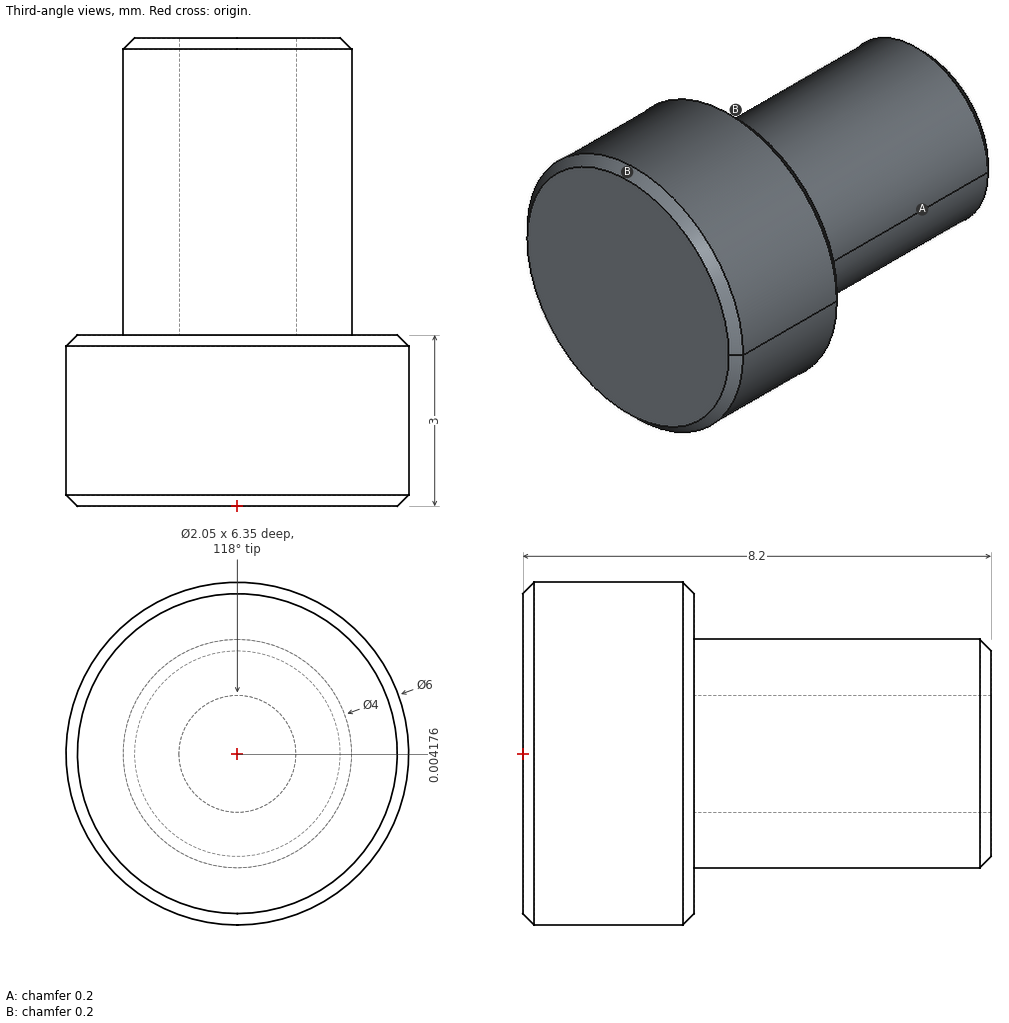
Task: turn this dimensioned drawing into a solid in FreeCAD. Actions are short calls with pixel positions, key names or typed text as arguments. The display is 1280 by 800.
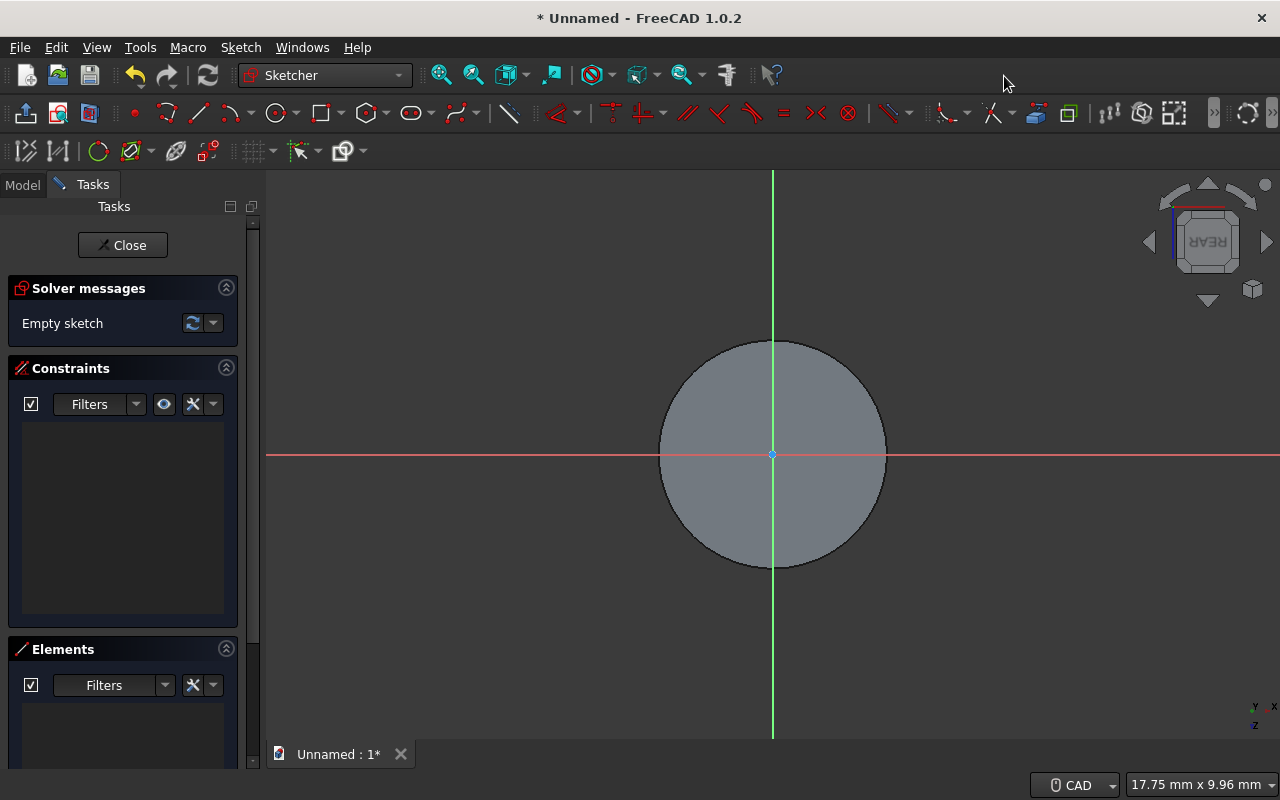
scroll(802, 454, up, 6)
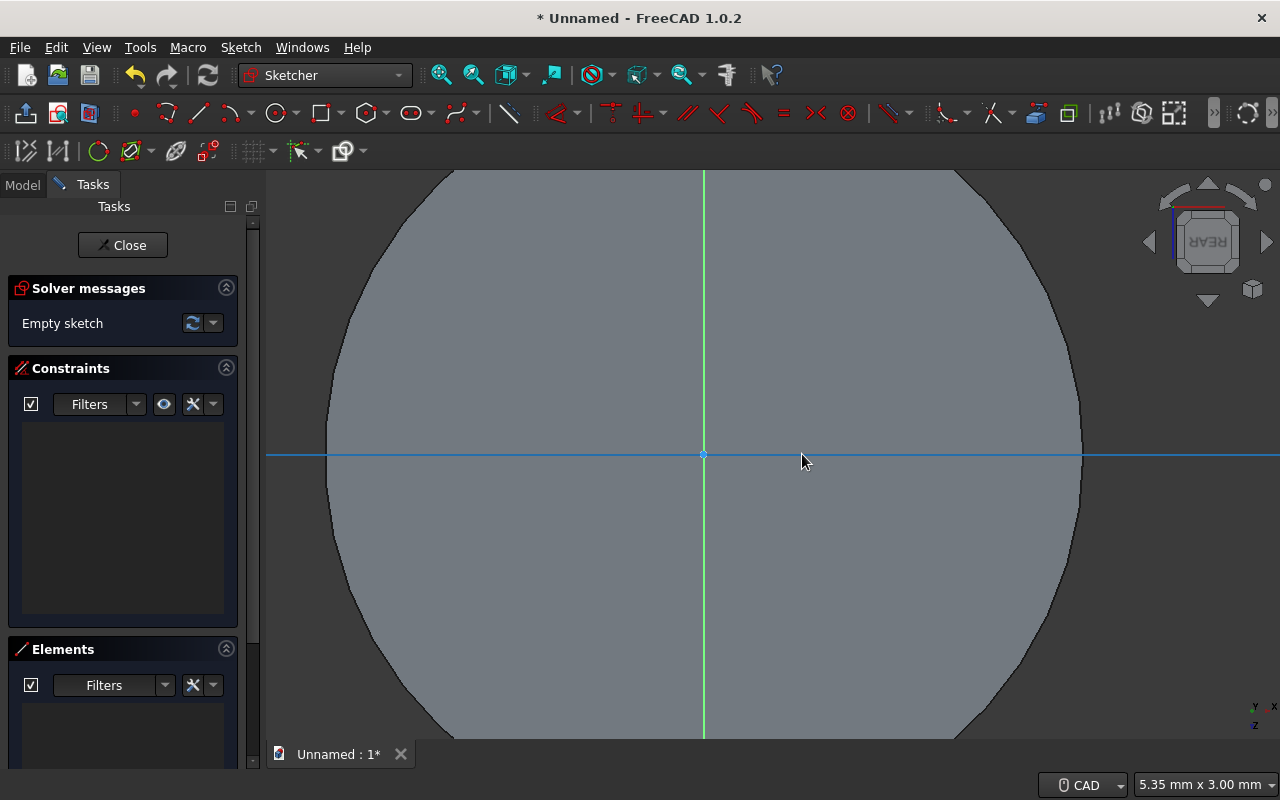
click(276, 114)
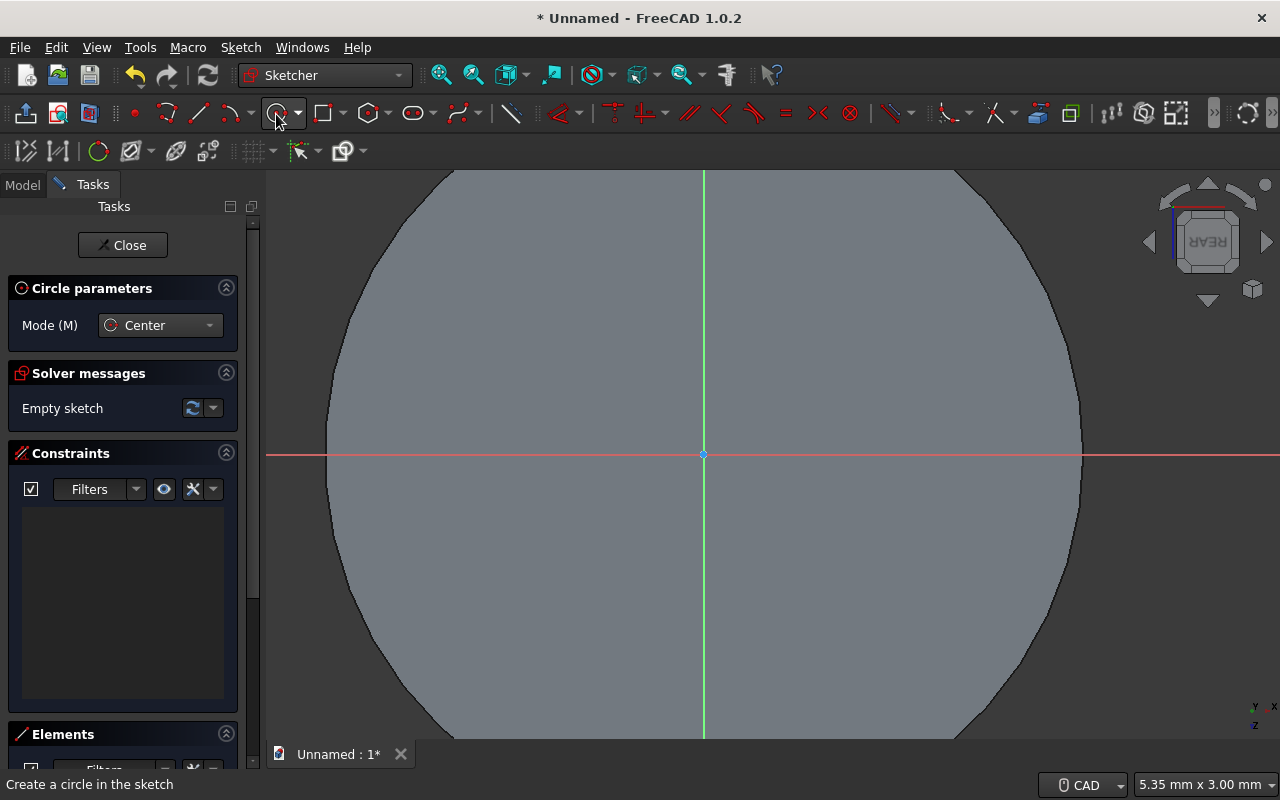
scroll(704, 454, up, 15)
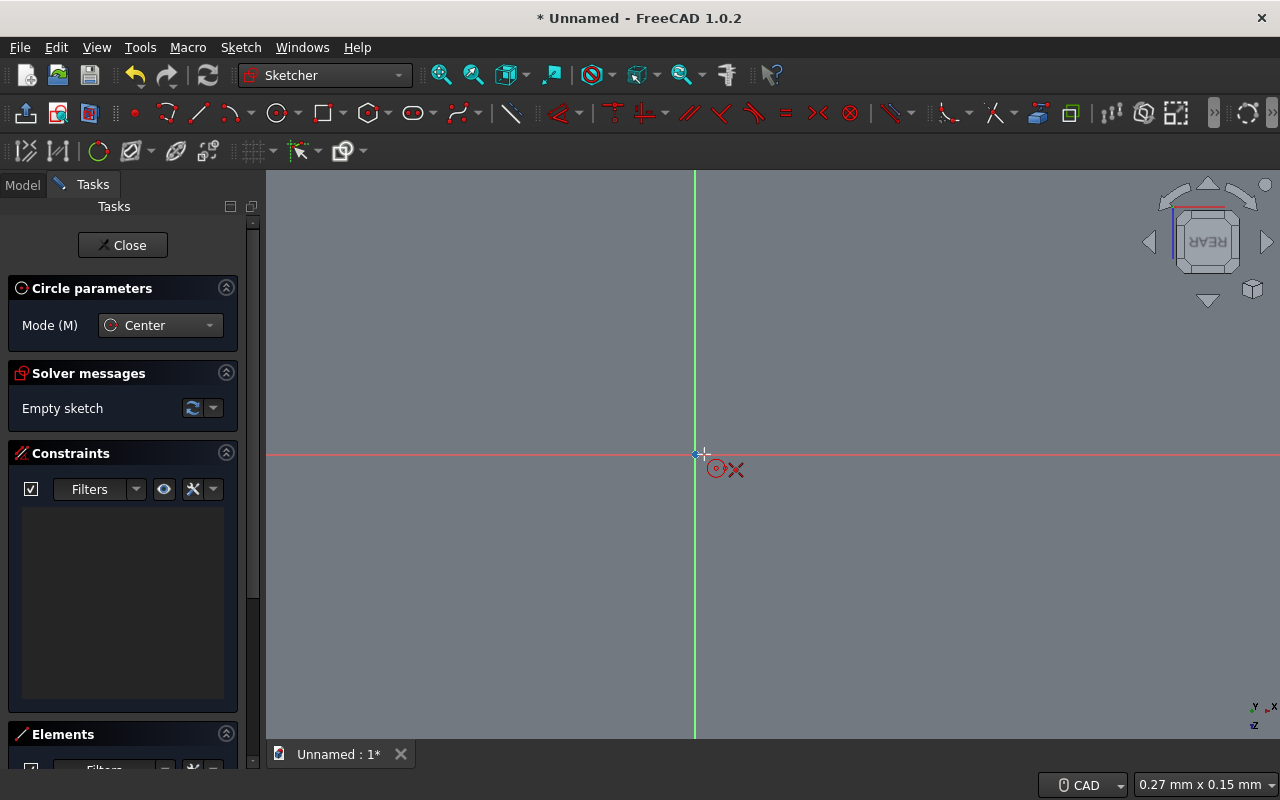
click(695, 439)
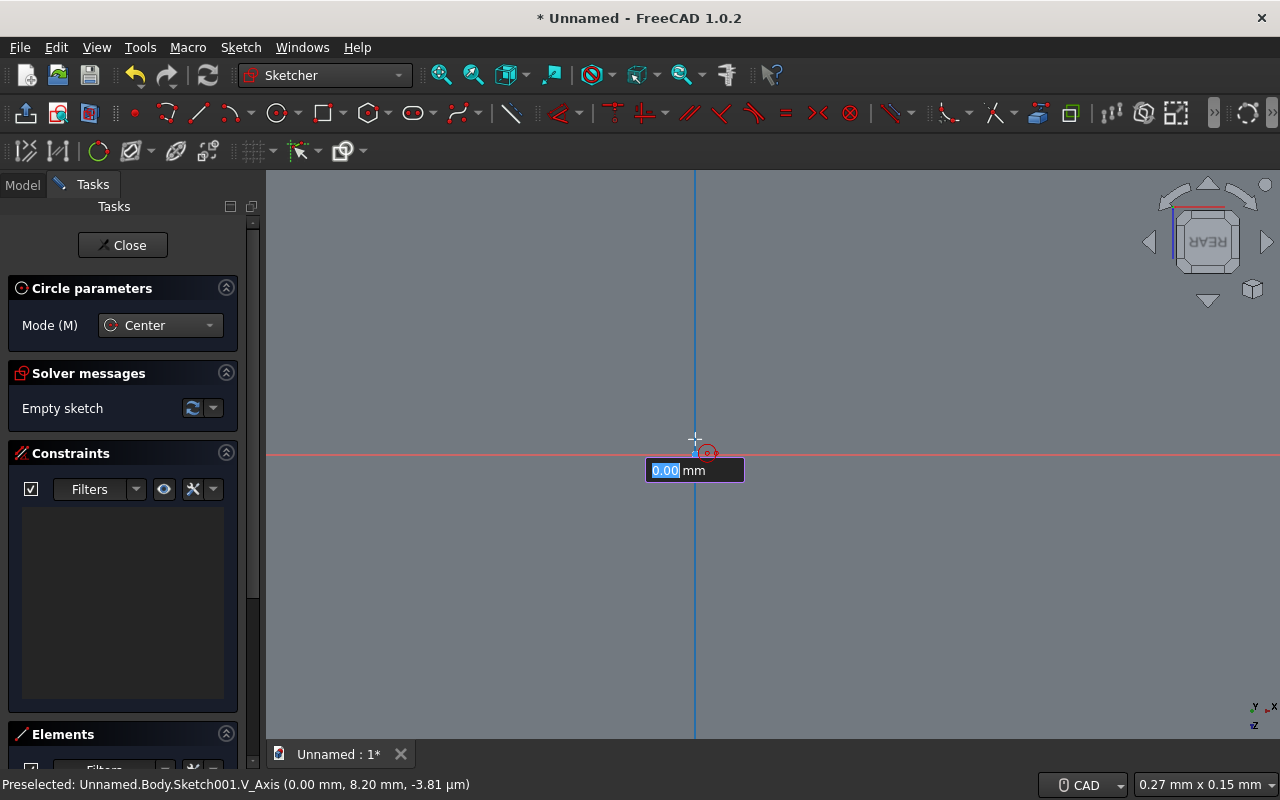
scroll(705, 455, down, 15)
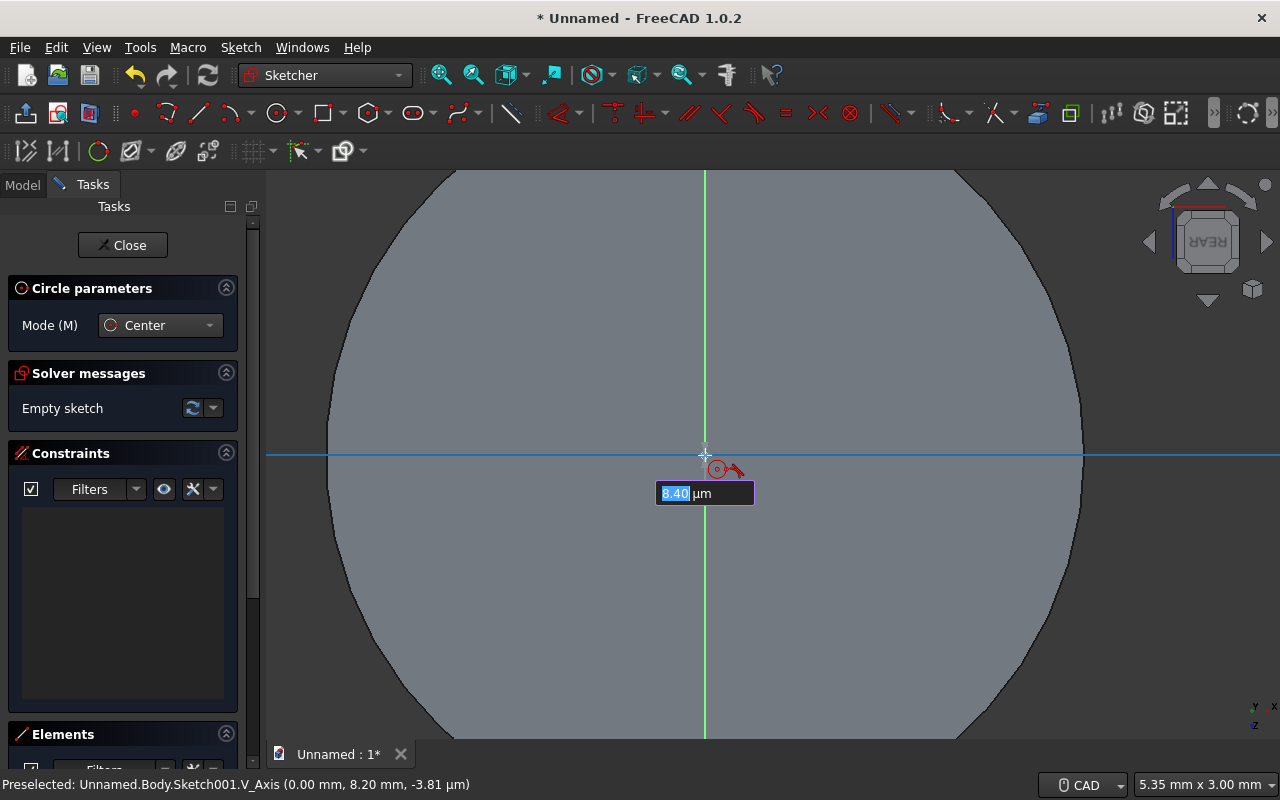
click(842, 317)
key(Escape)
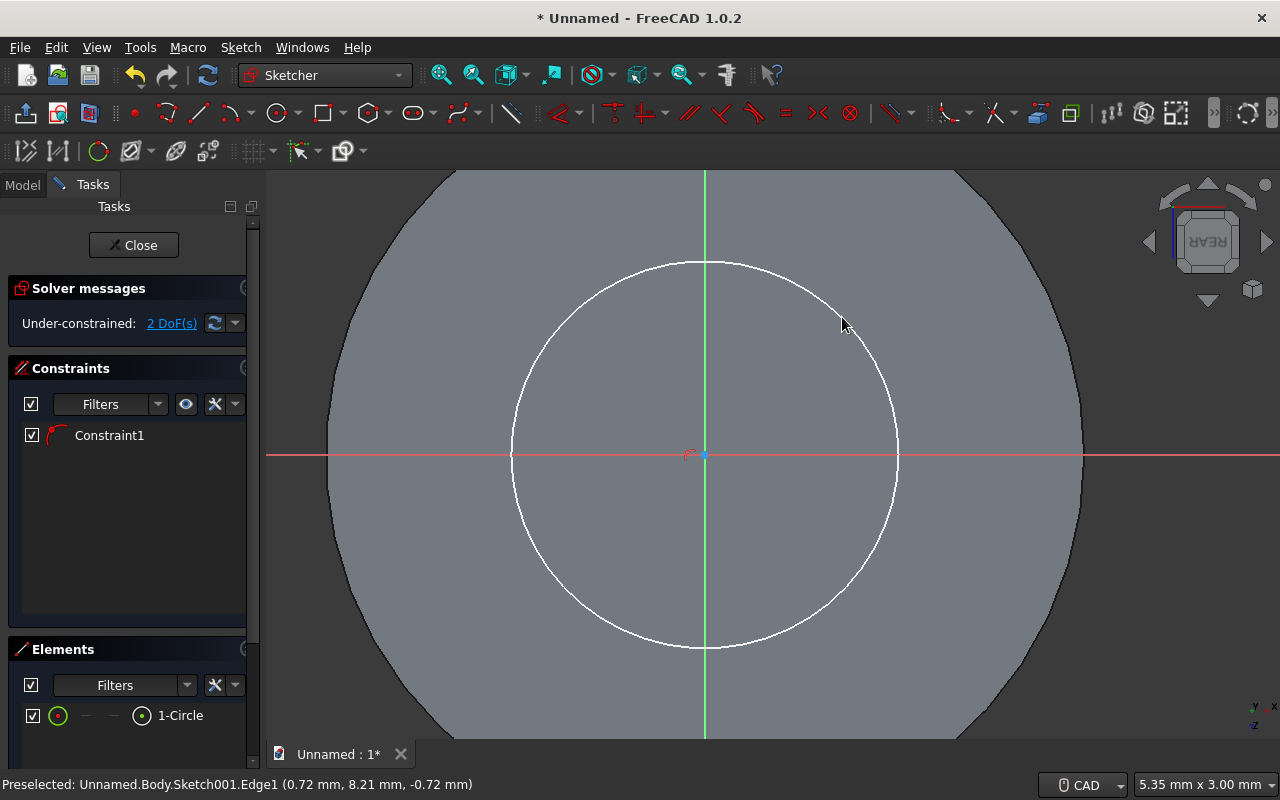
click(558, 114)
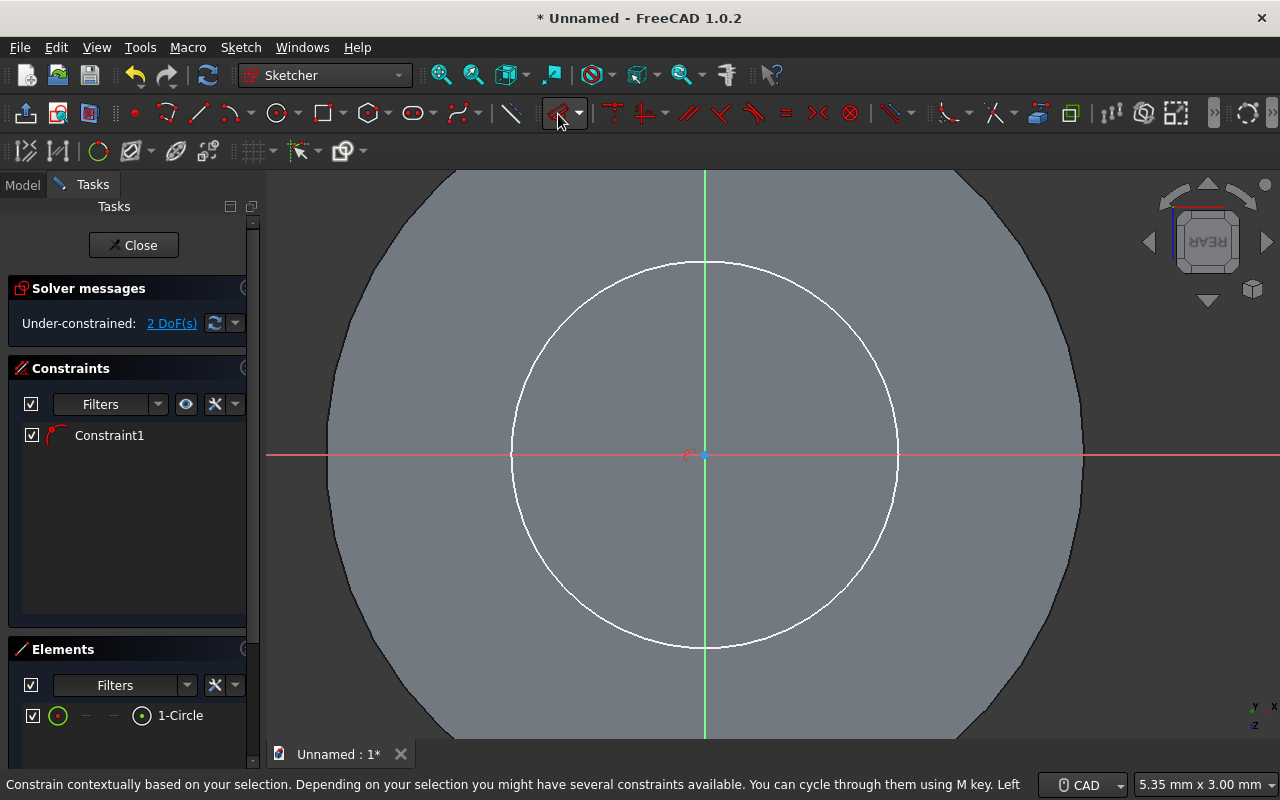
click(841, 317)
click(863, 294)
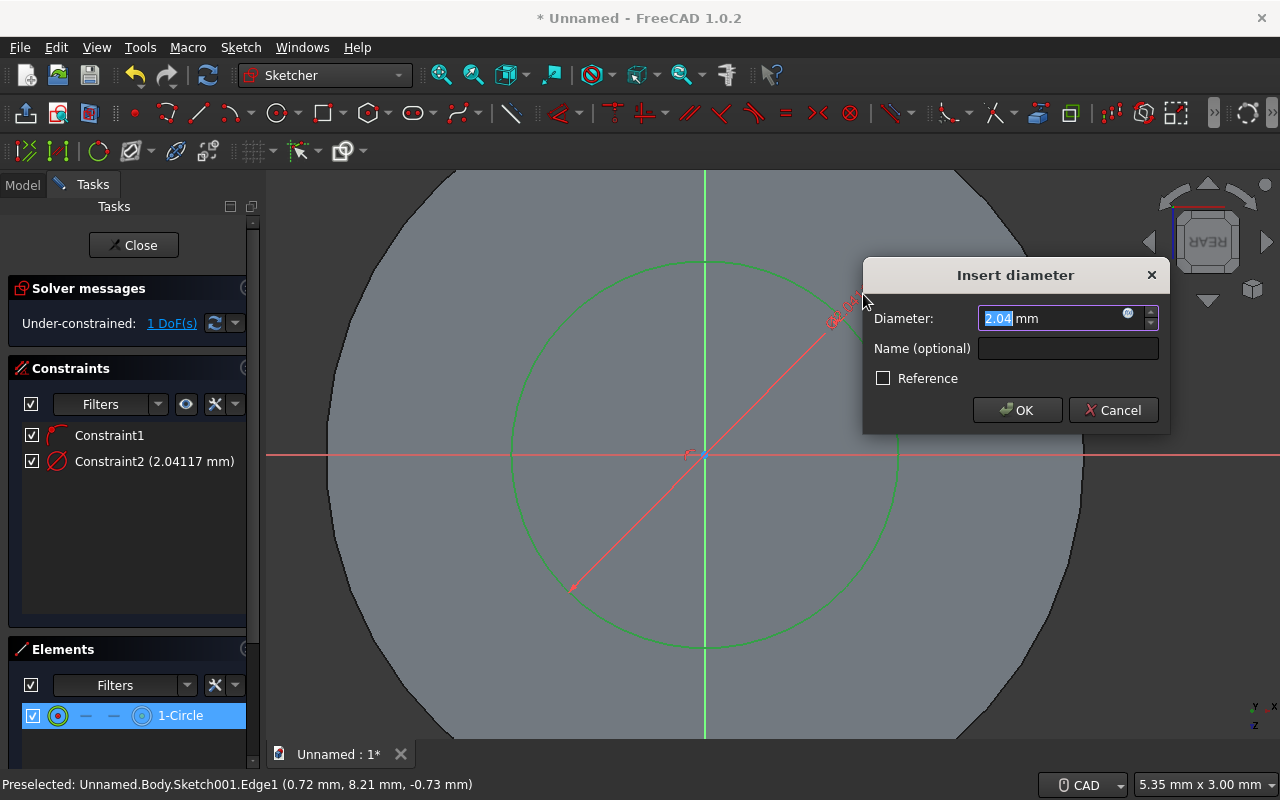
text(2.05)
key(Return)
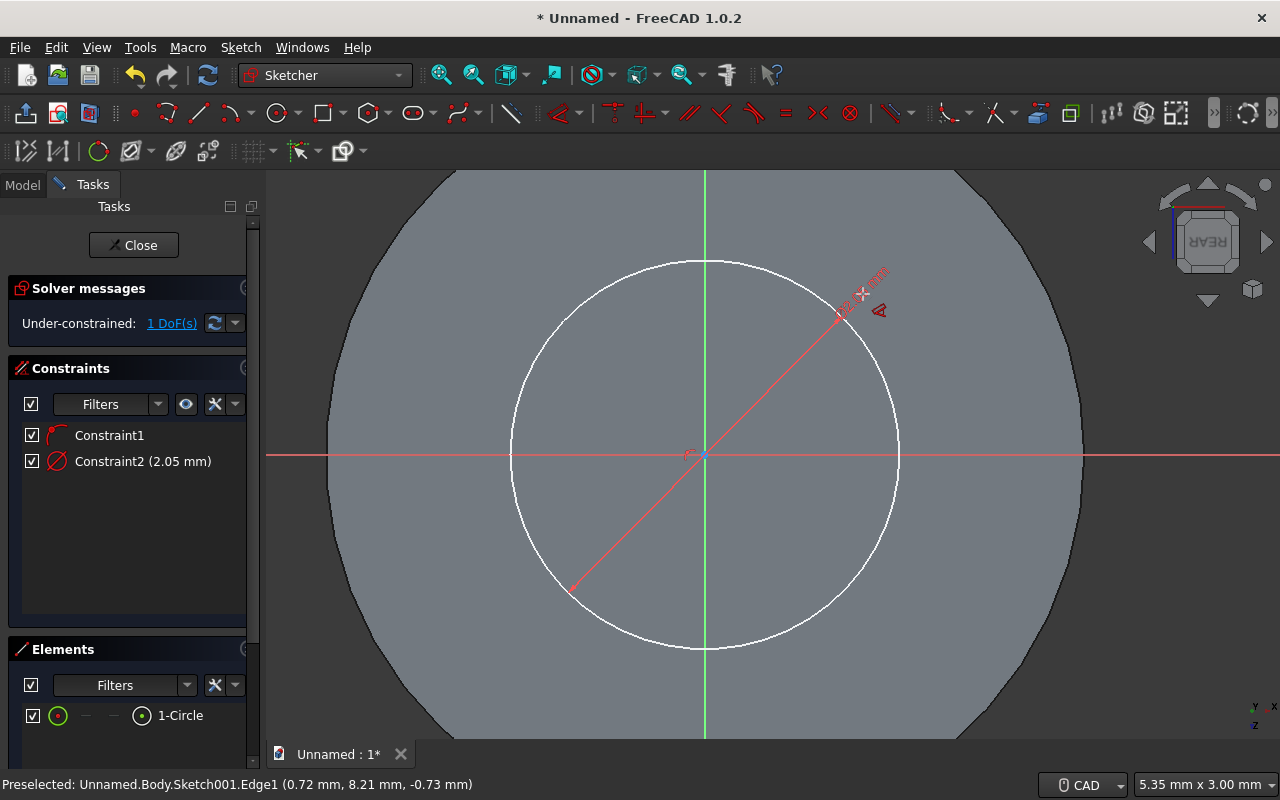
scroll(705, 455, up, 20)